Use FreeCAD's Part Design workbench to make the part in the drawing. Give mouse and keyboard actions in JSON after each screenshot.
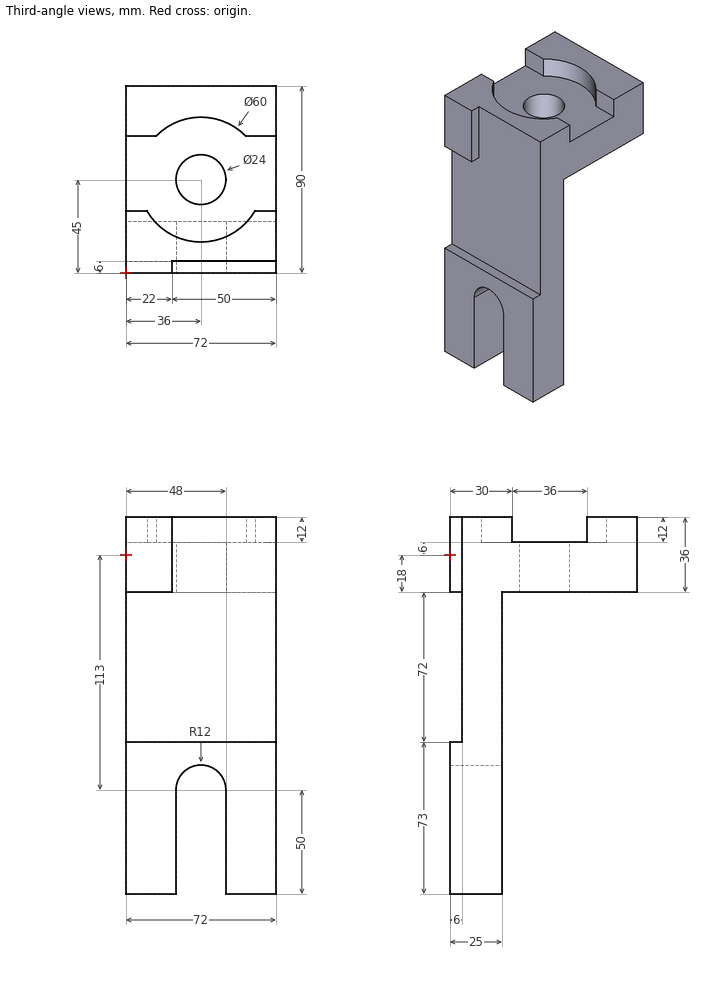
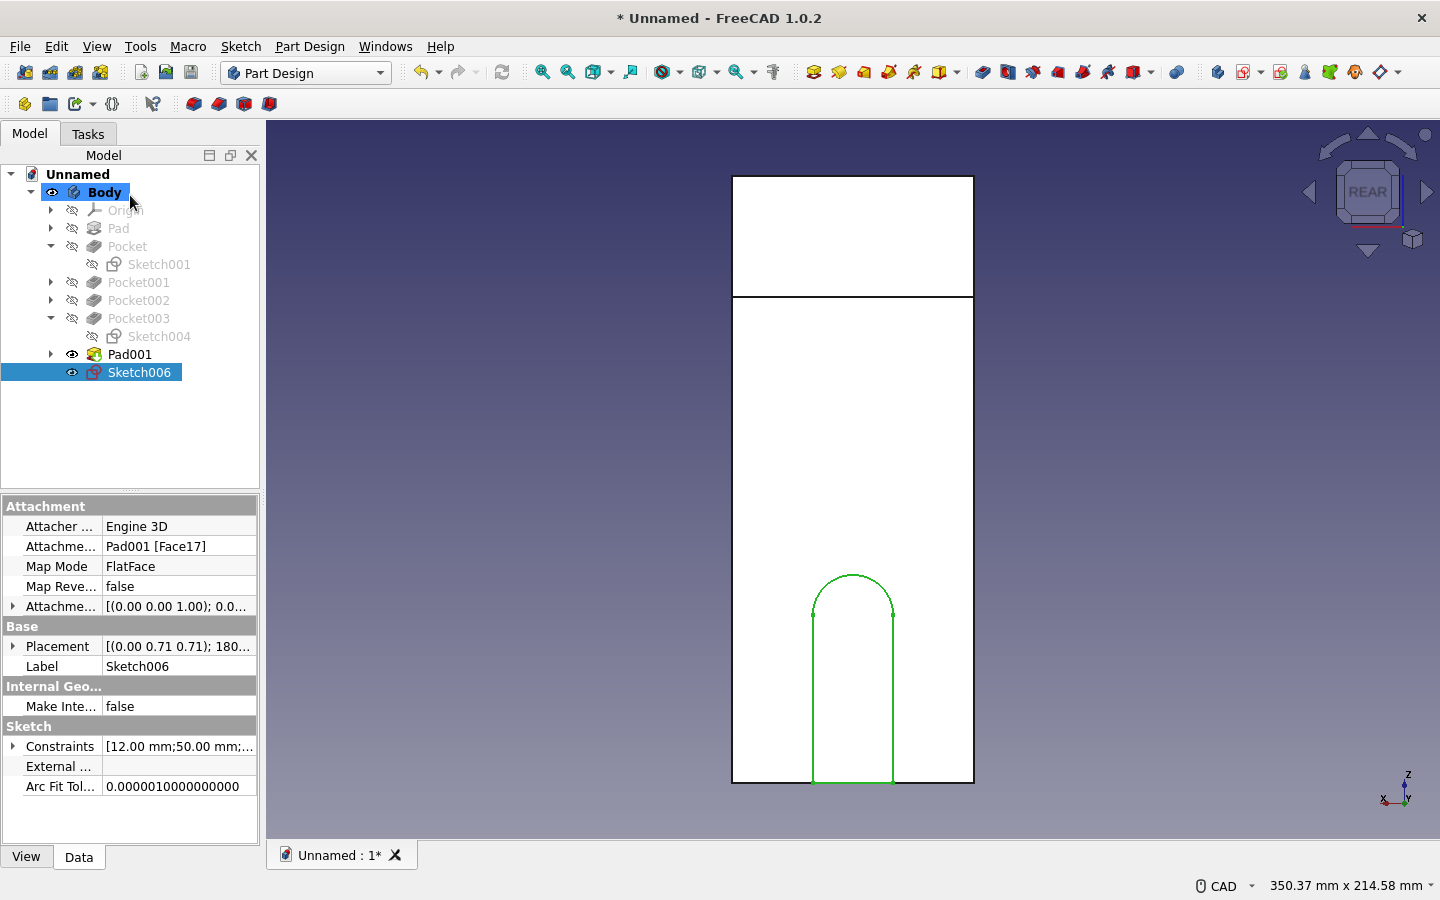
{"action": "left_click", "coordinate": [983, 72]}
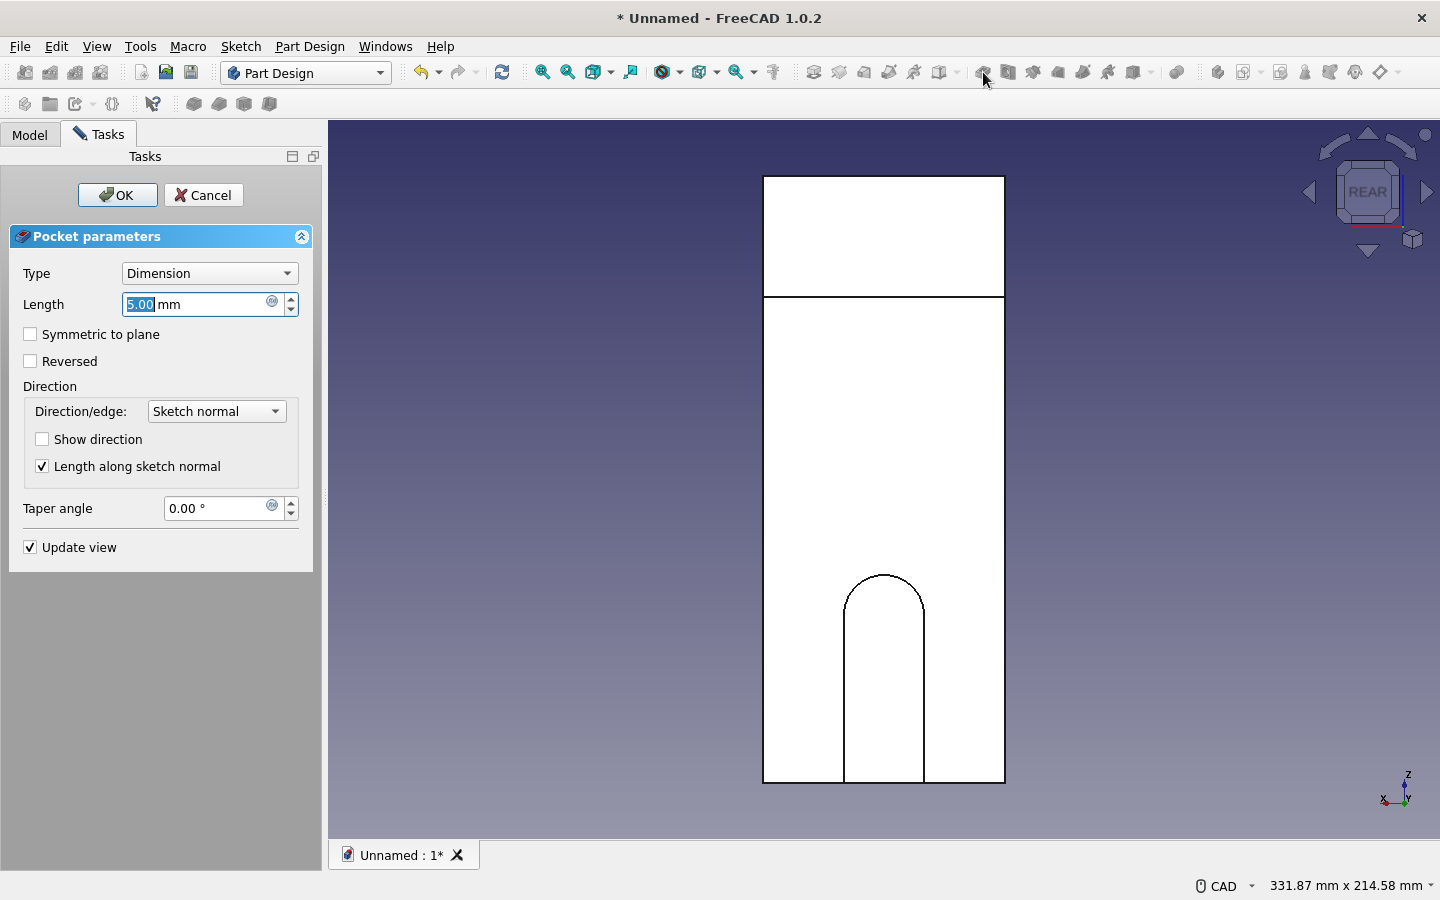
{"action": "left_click", "coordinate": [210, 274]}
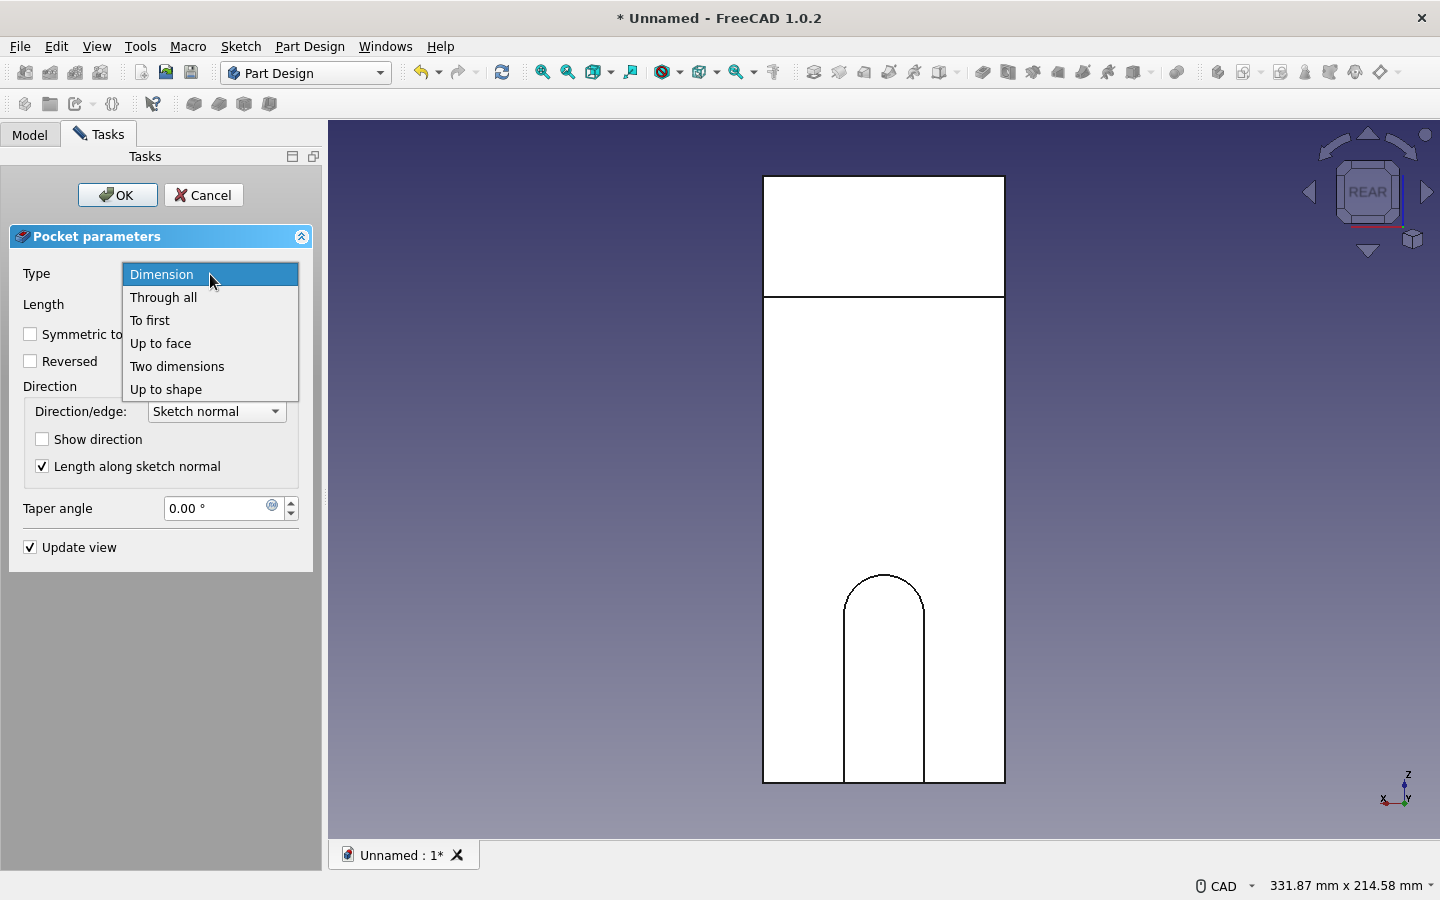
{"action": "left_click", "coordinate": [208, 298]}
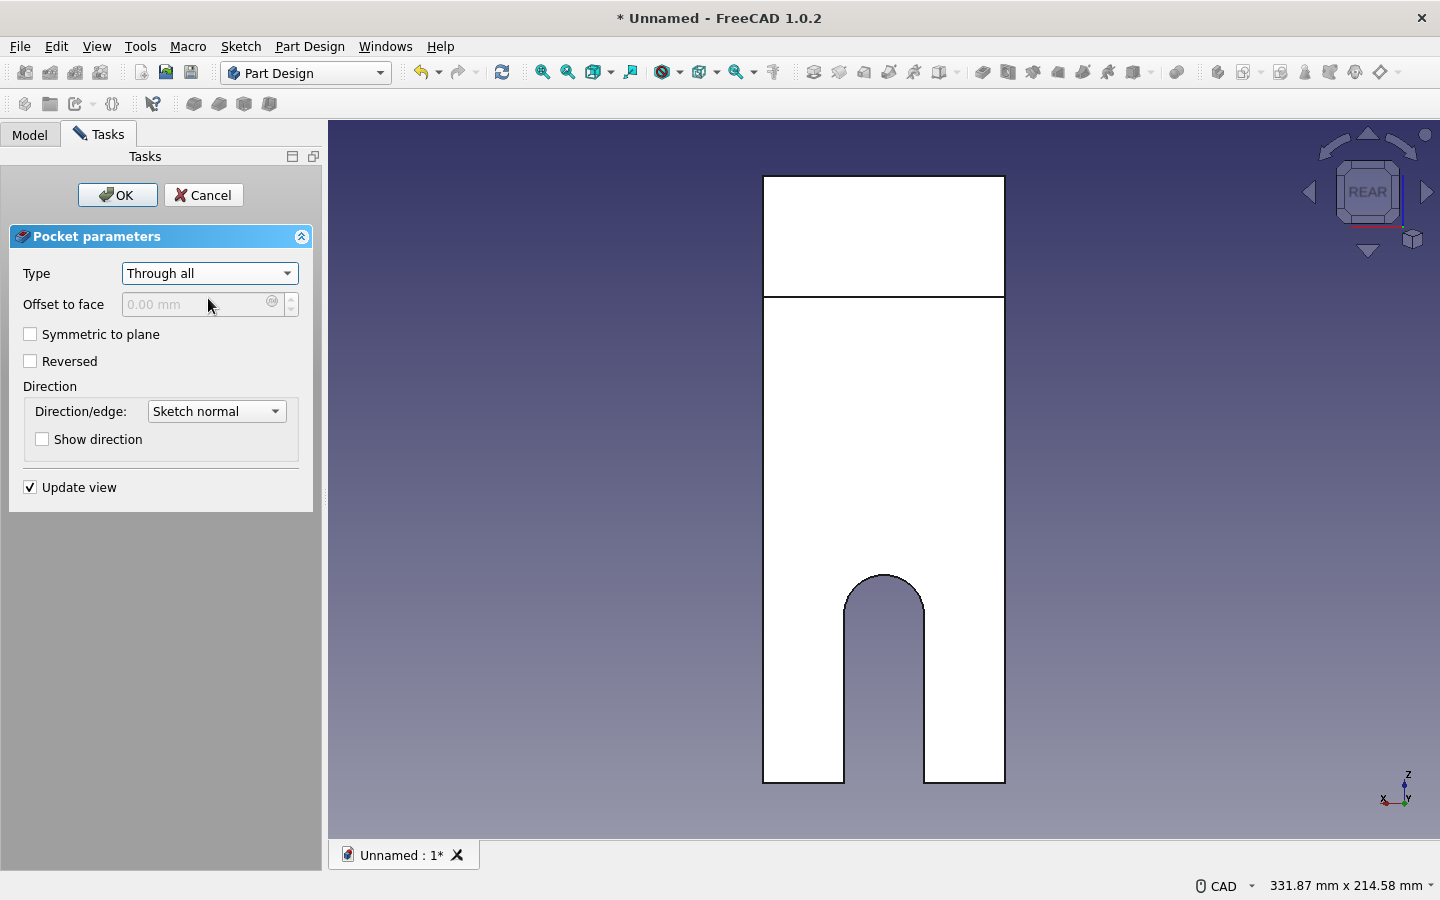
{"action": "left_click", "coordinate": [118, 195]}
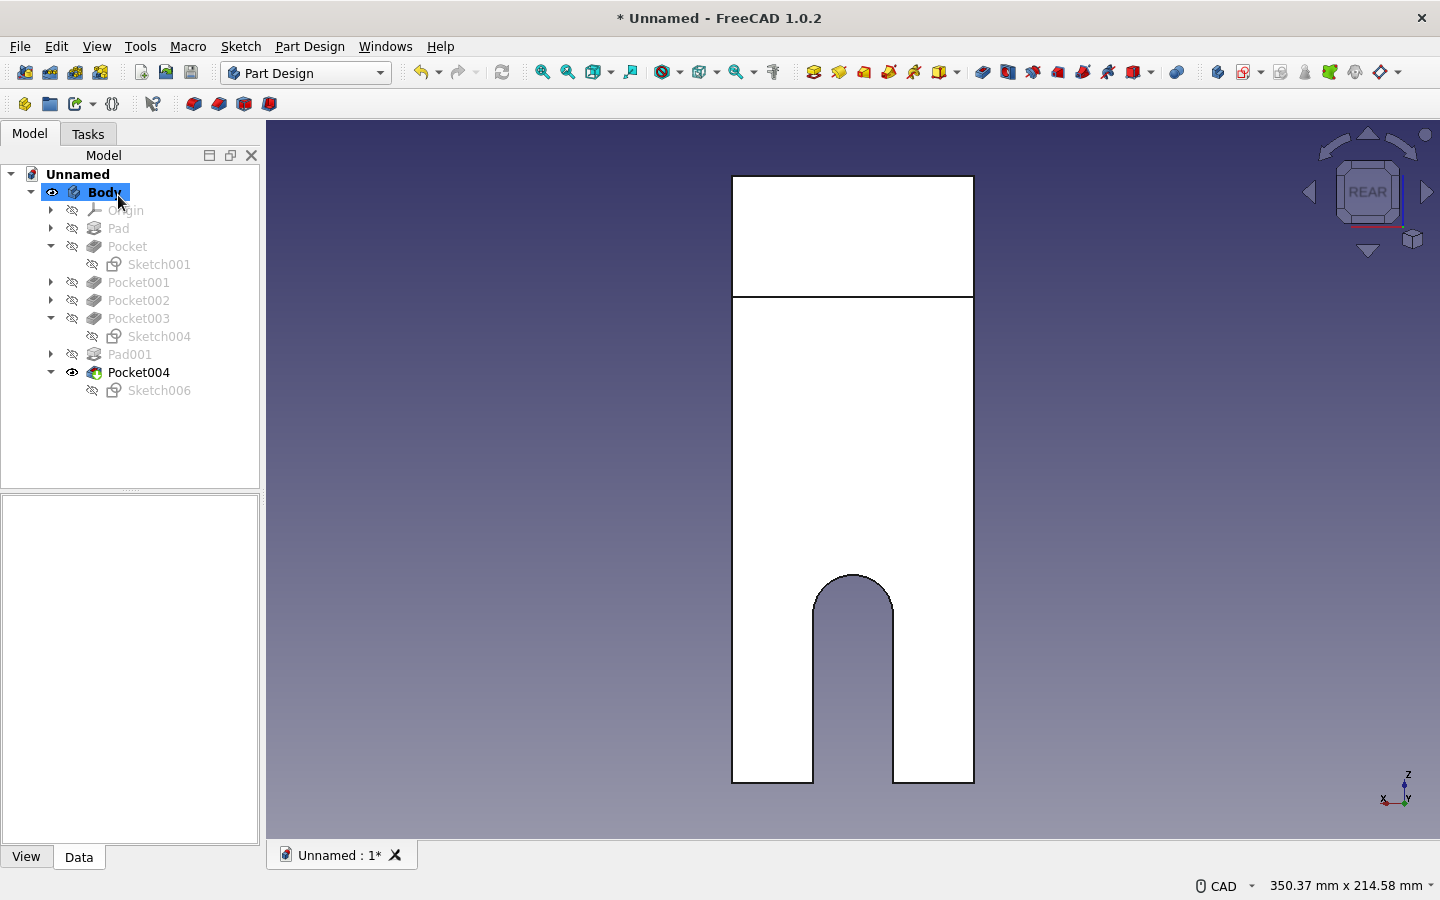
{"action": "key", "text": "0"}